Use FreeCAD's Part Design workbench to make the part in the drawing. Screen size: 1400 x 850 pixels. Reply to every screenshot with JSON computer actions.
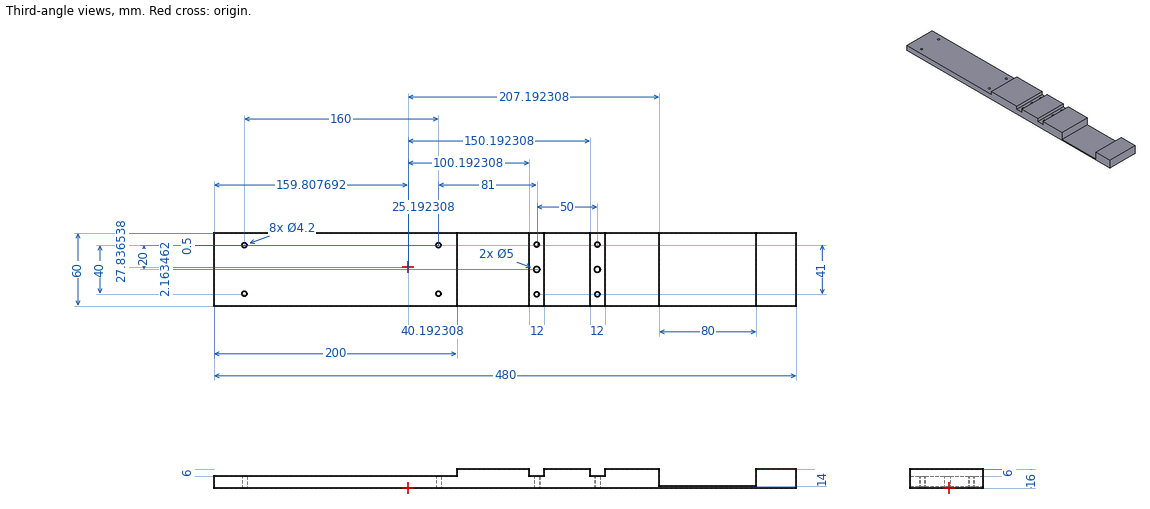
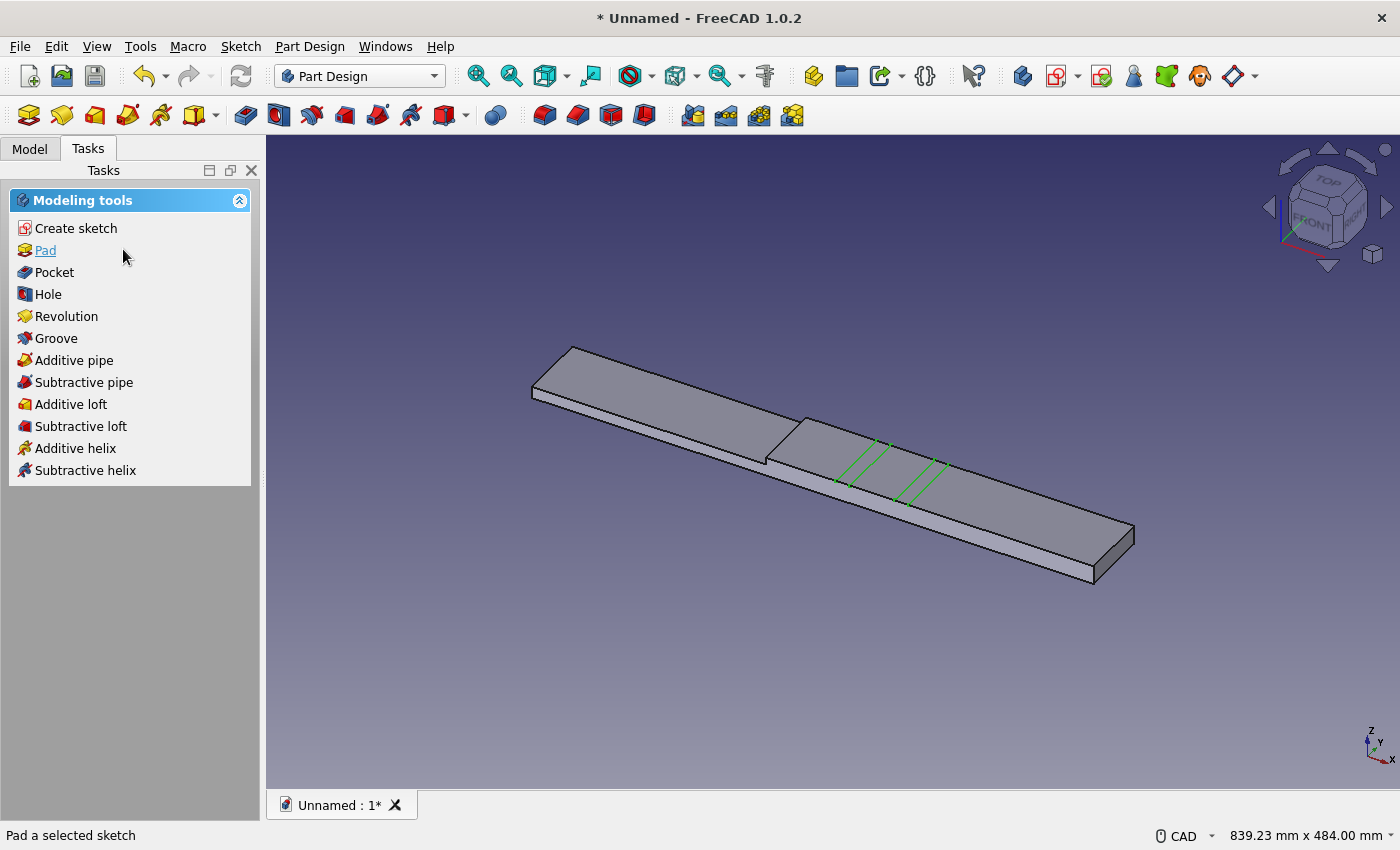
{"action": "left_click", "coordinate": [246, 116]}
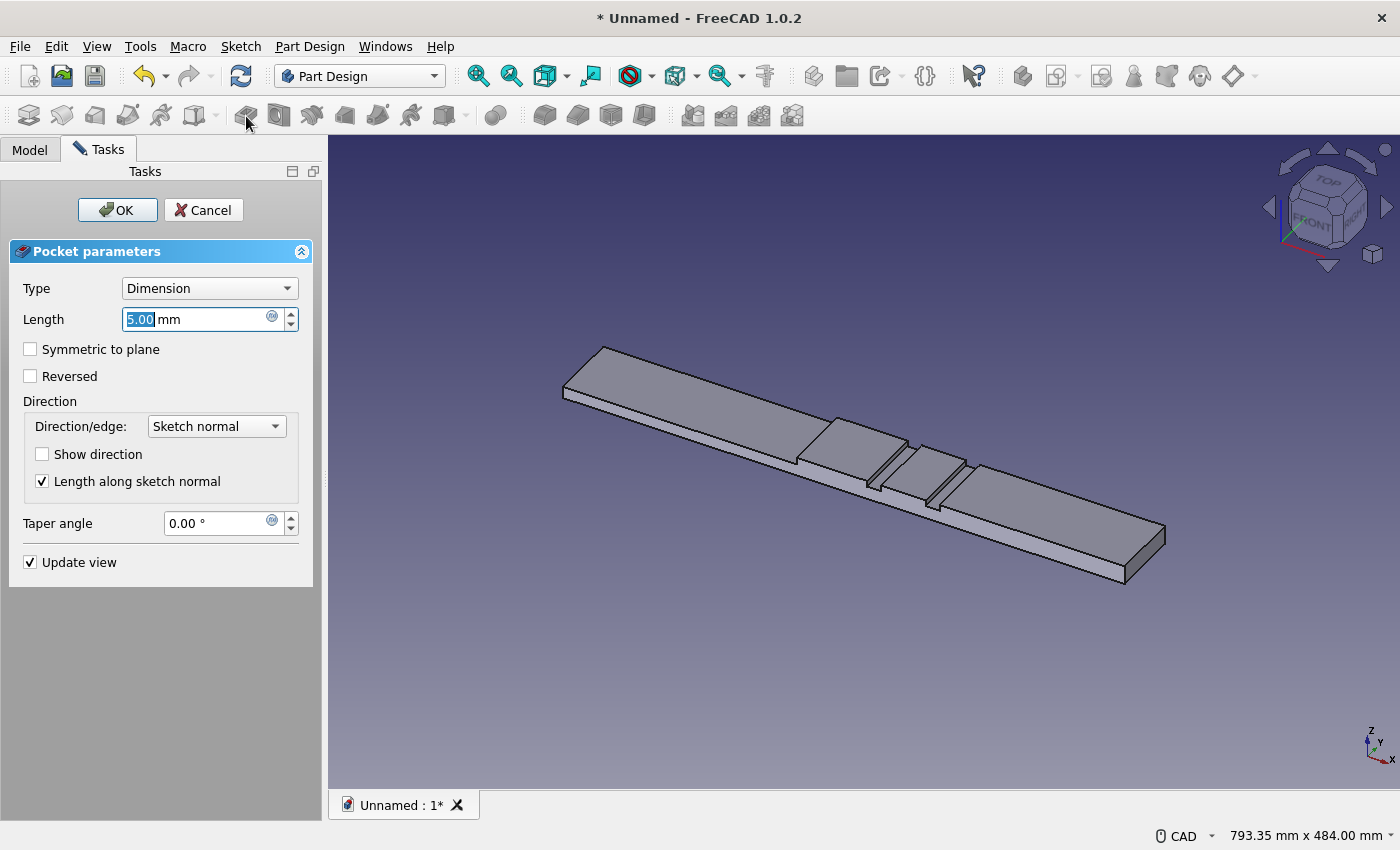
{"action": "type", "text": "6"}
{"action": "key", "text": "Tab"}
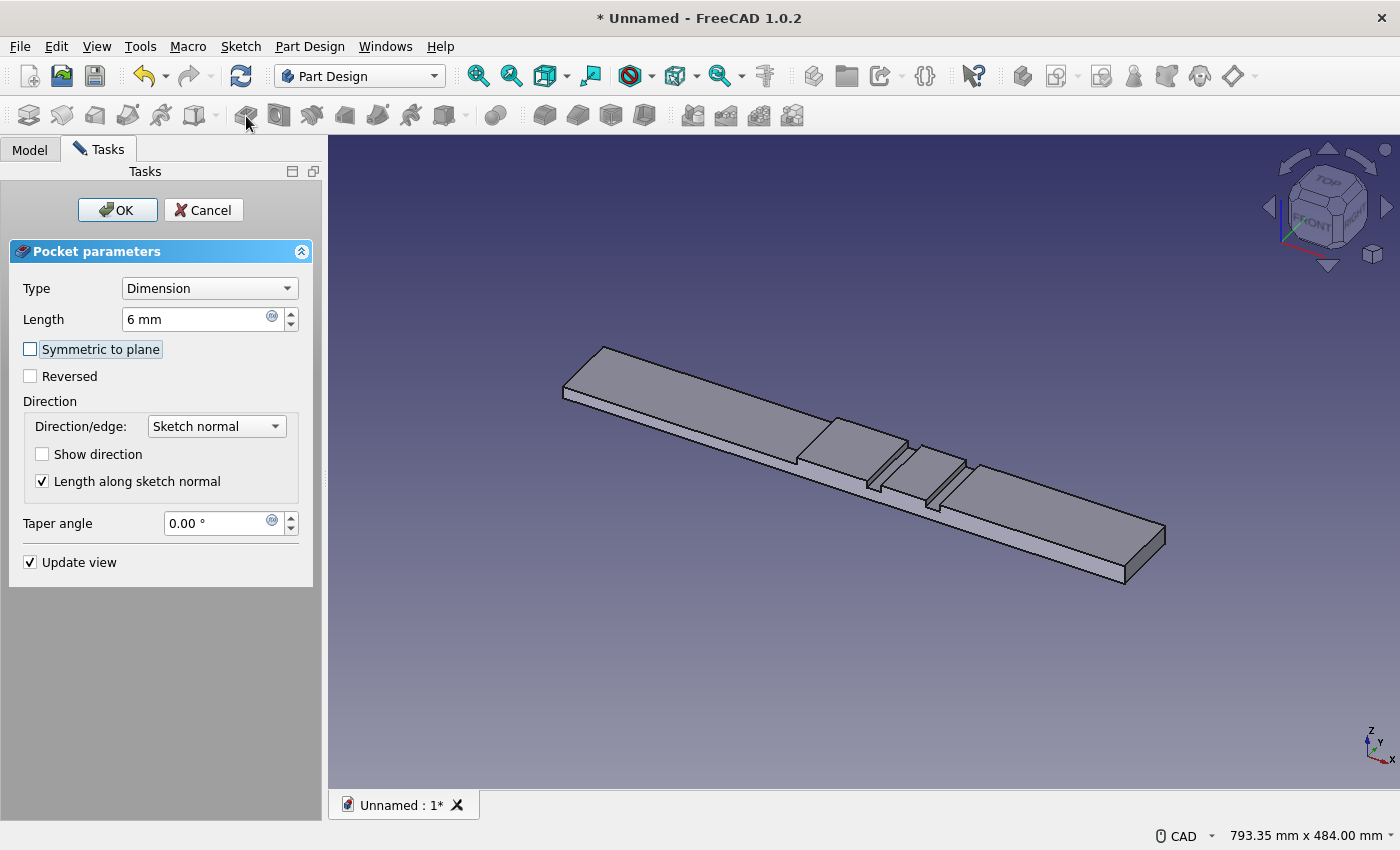
{"action": "left_click", "coordinate": [118, 210]}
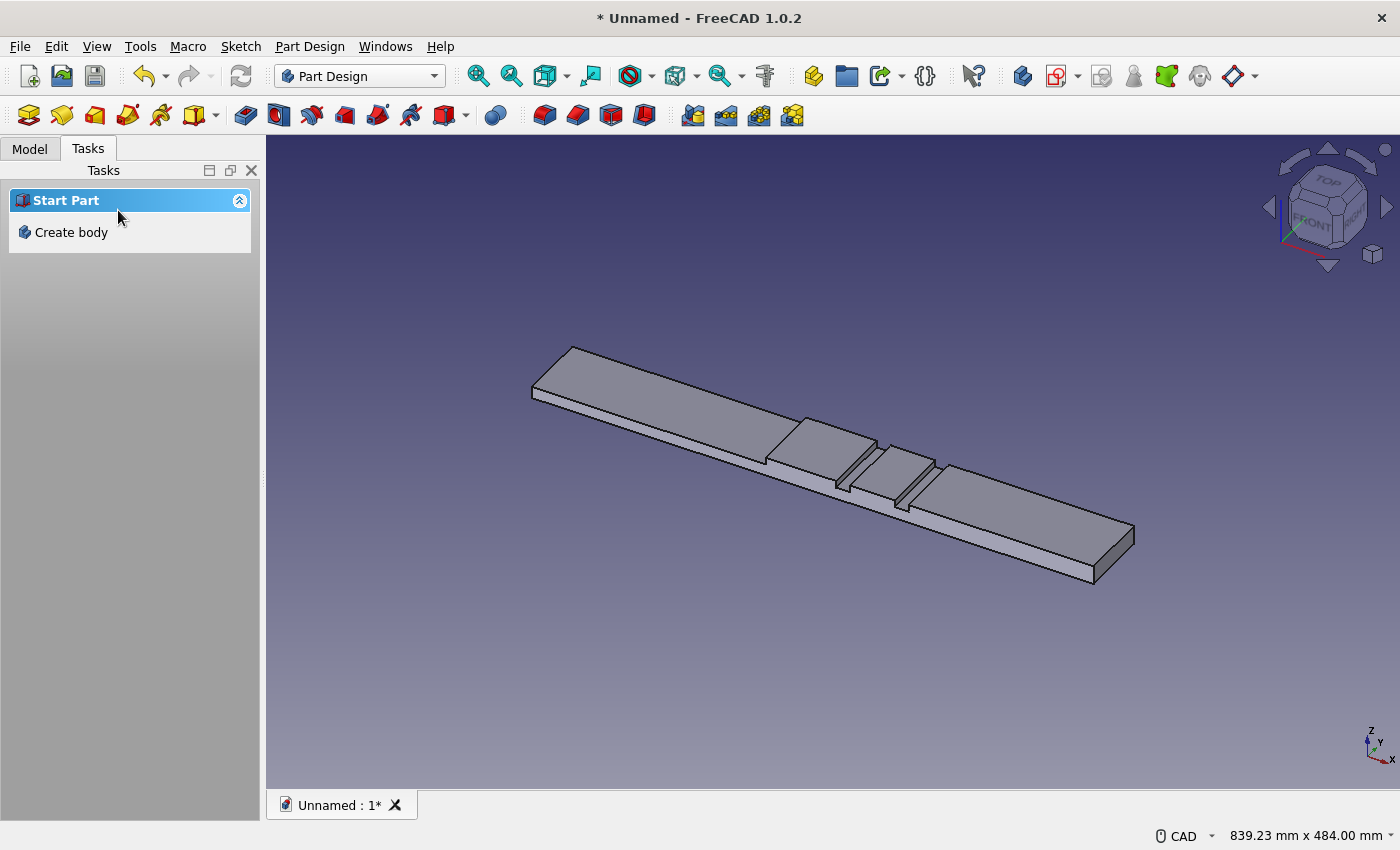
{"action": "left_click", "coordinate": [736, 427]}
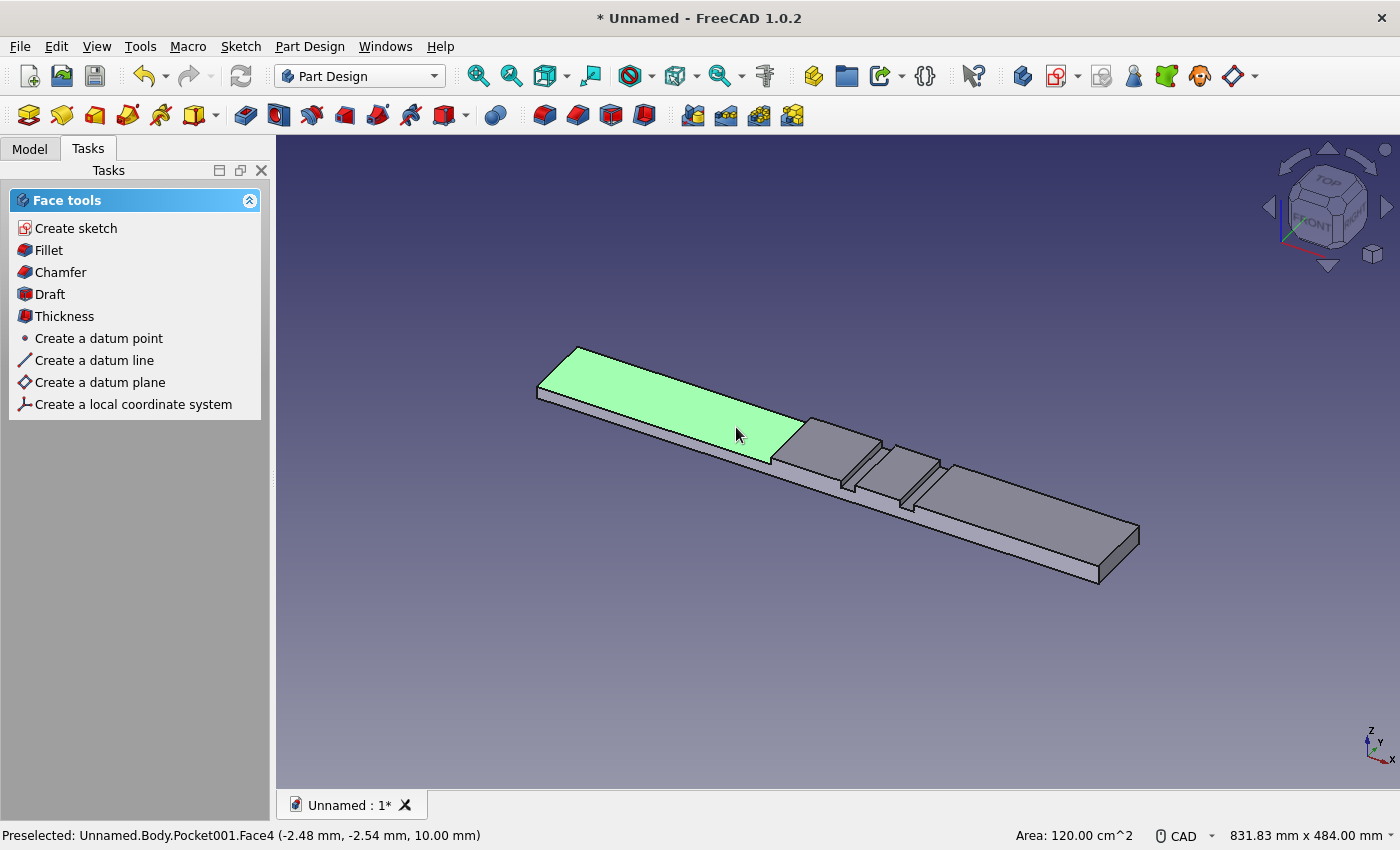
{"action": "left_click", "coordinate": [1056, 76]}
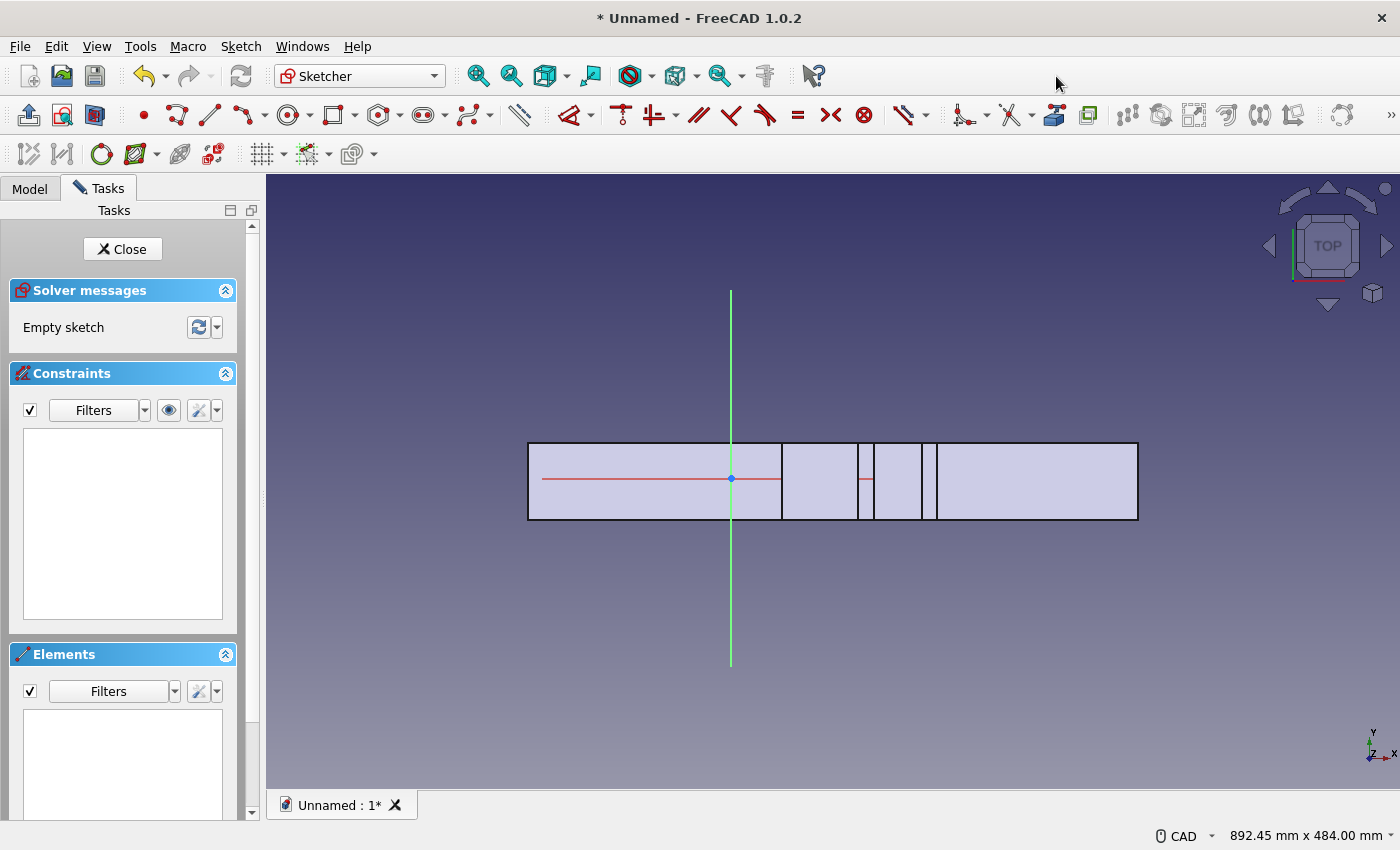
{"action": "left_click", "coordinate": [95, 116]}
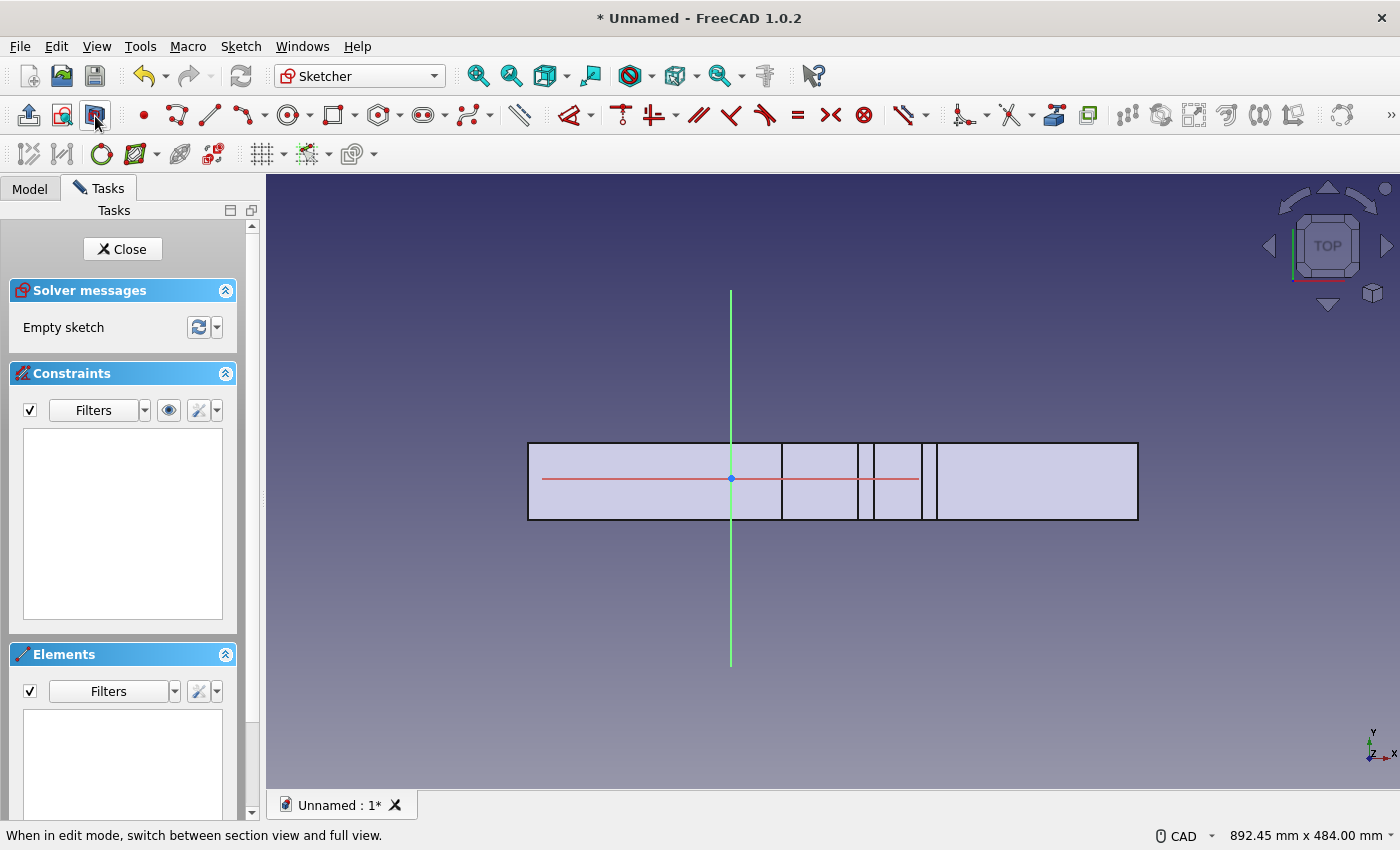
{"action": "scroll", "coordinate": [721, 482], "scroll_direction": "up", "scroll_amount": 3}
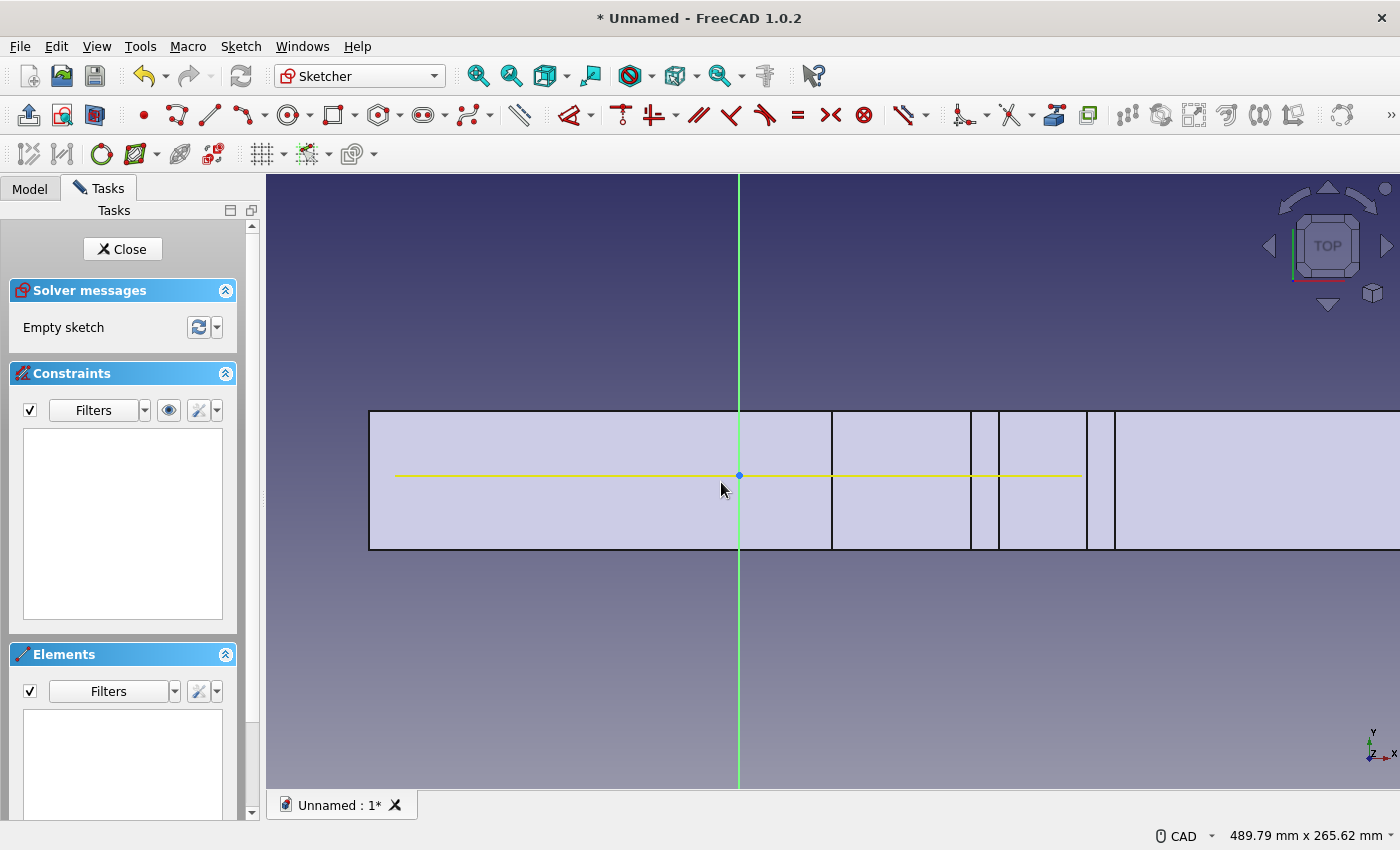
{"action": "left_click", "coordinate": [288, 116]}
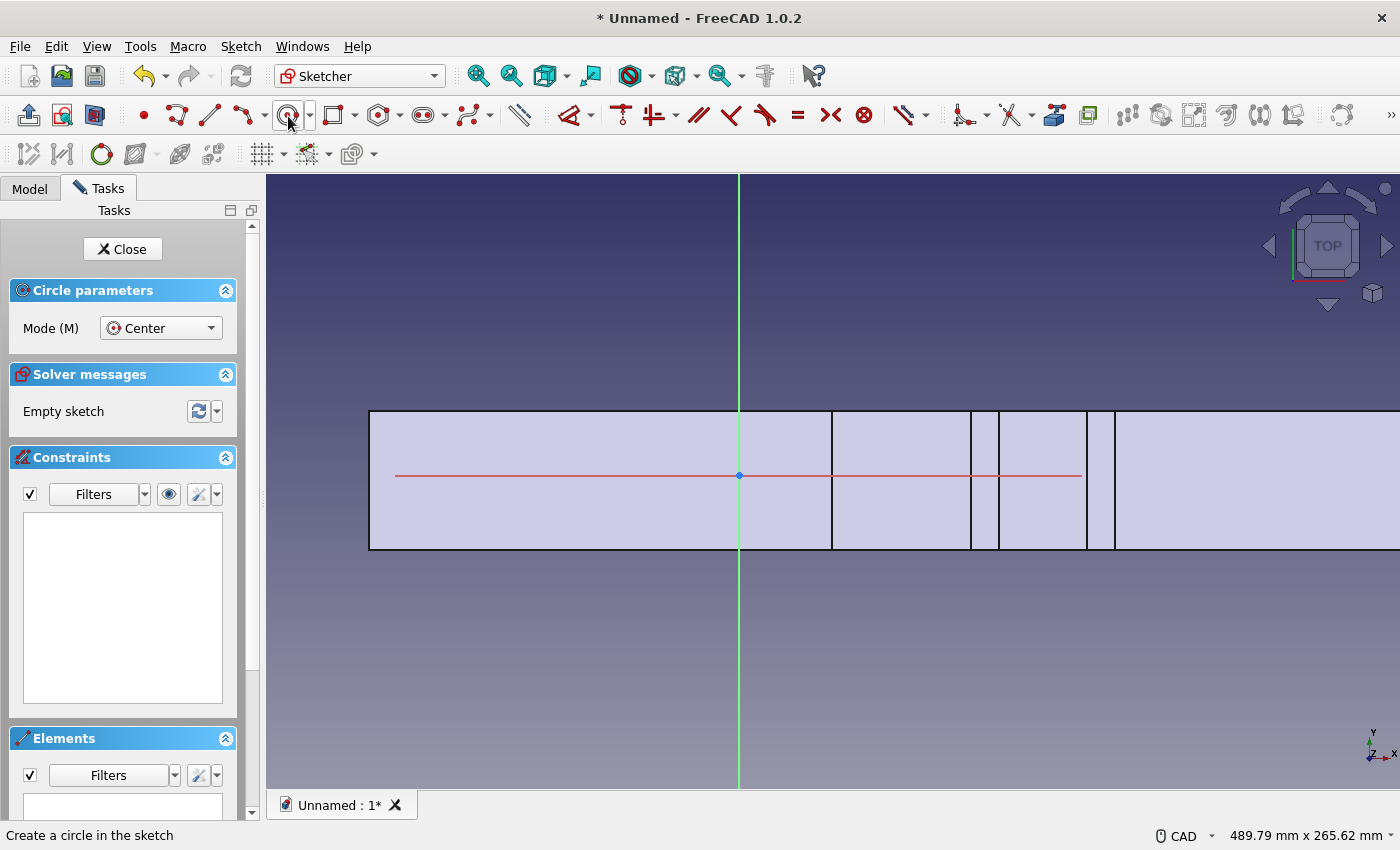
{"action": "scroll", "coordinate": [427, 434], "scroll_direction": "up", "scroll_amount": 8}